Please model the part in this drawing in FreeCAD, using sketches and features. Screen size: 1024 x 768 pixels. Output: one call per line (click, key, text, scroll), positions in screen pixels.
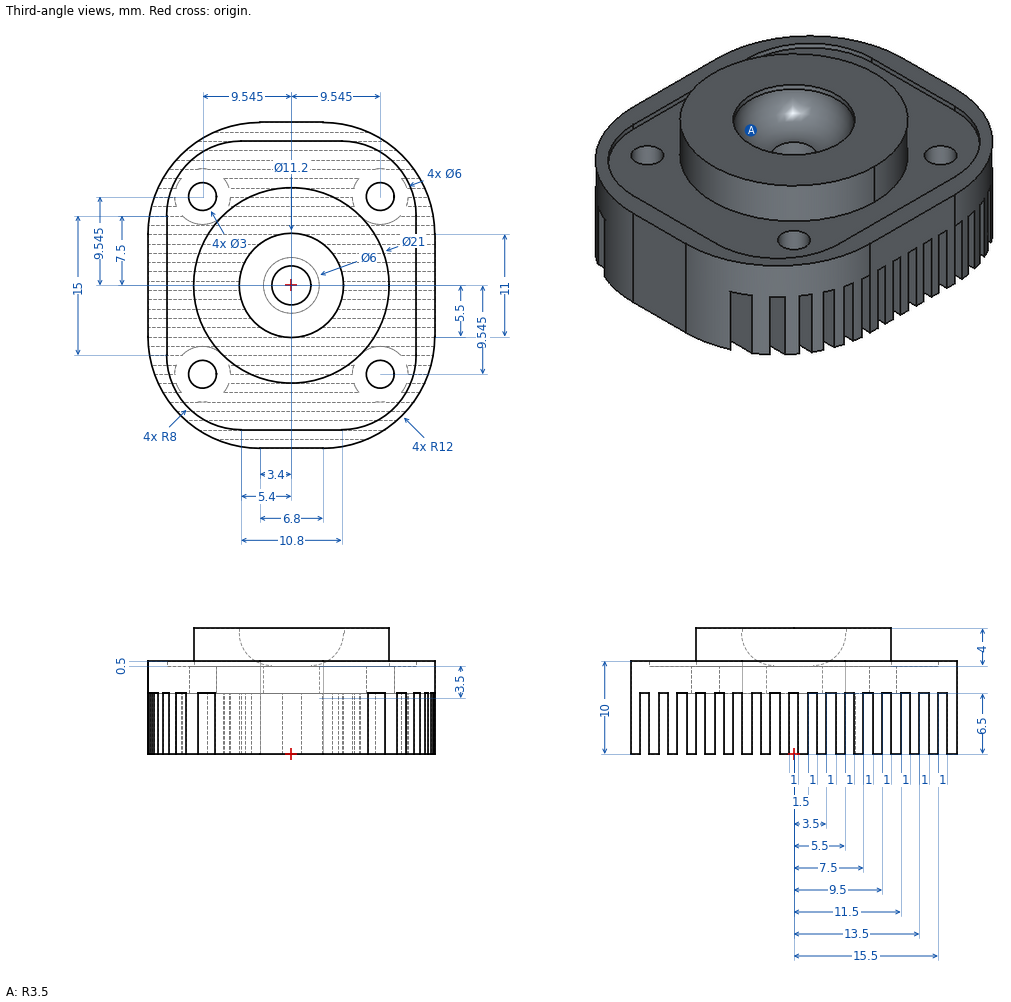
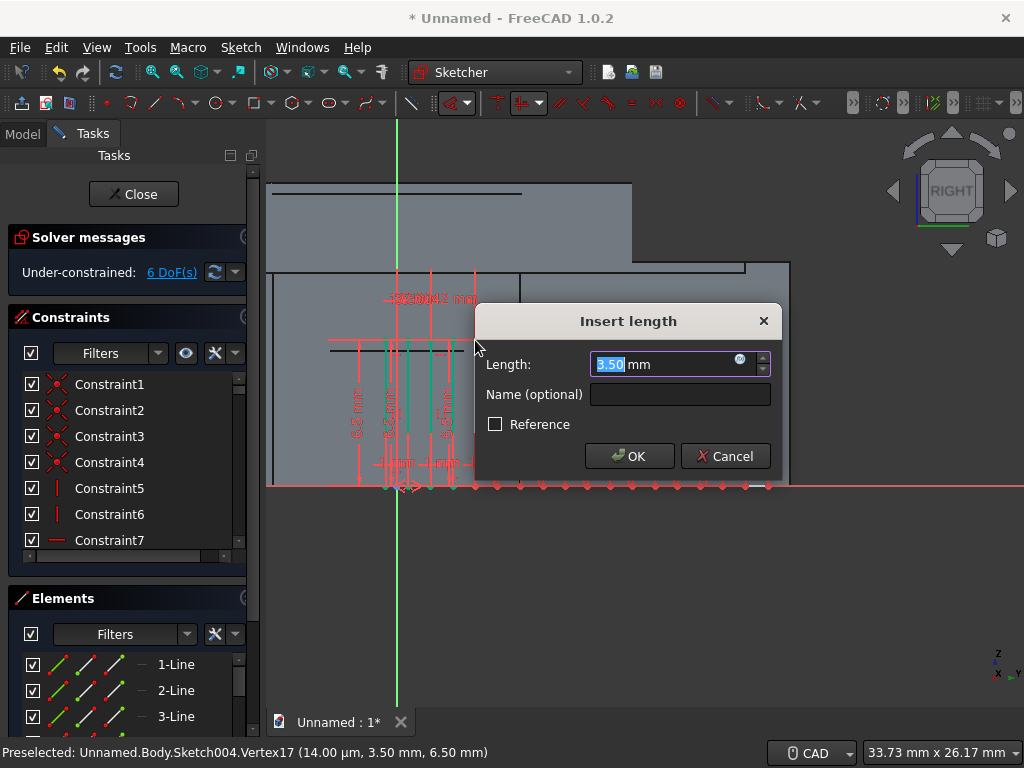
text(3.5)
key(Return)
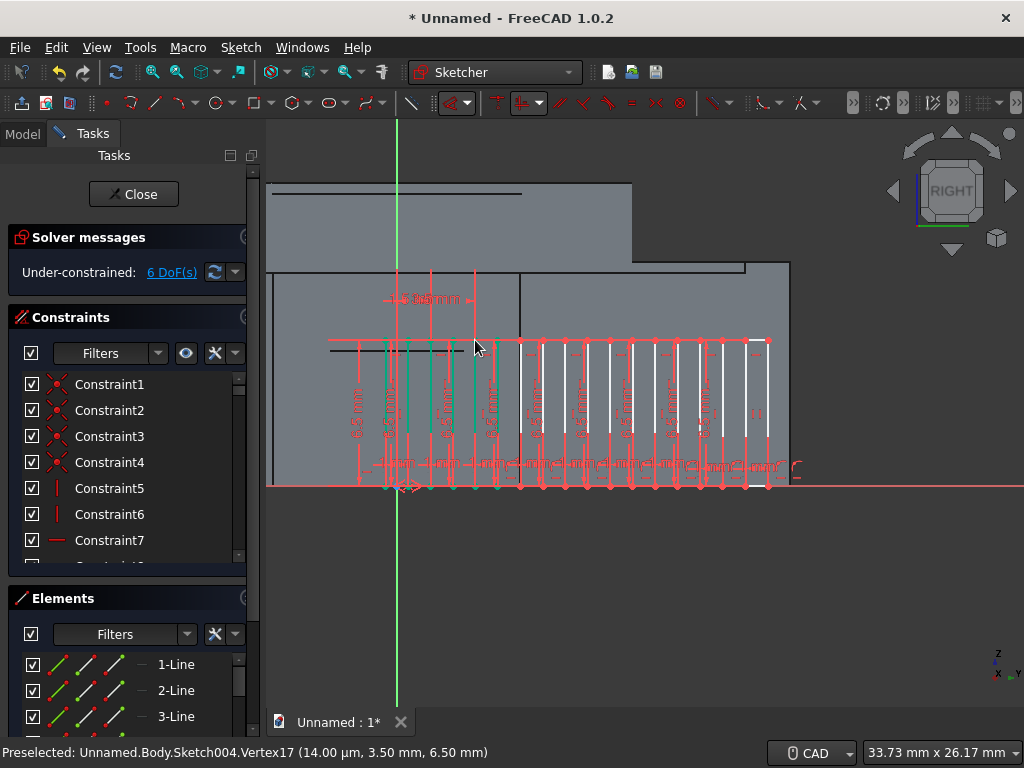
click(521, 340)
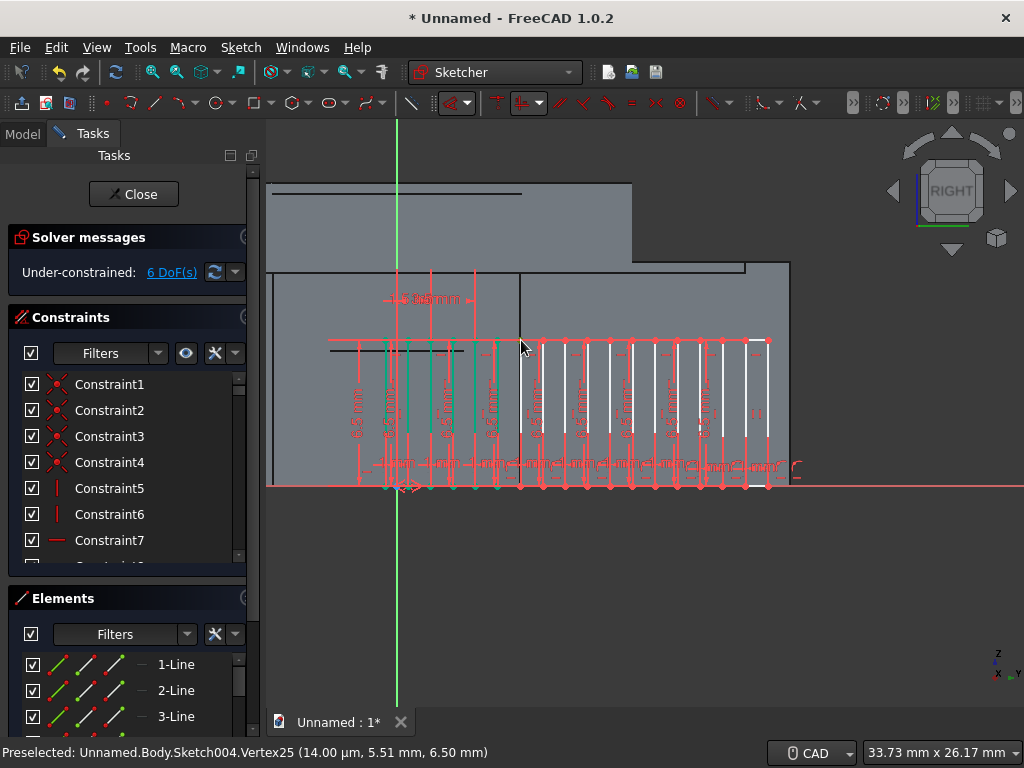
key(l)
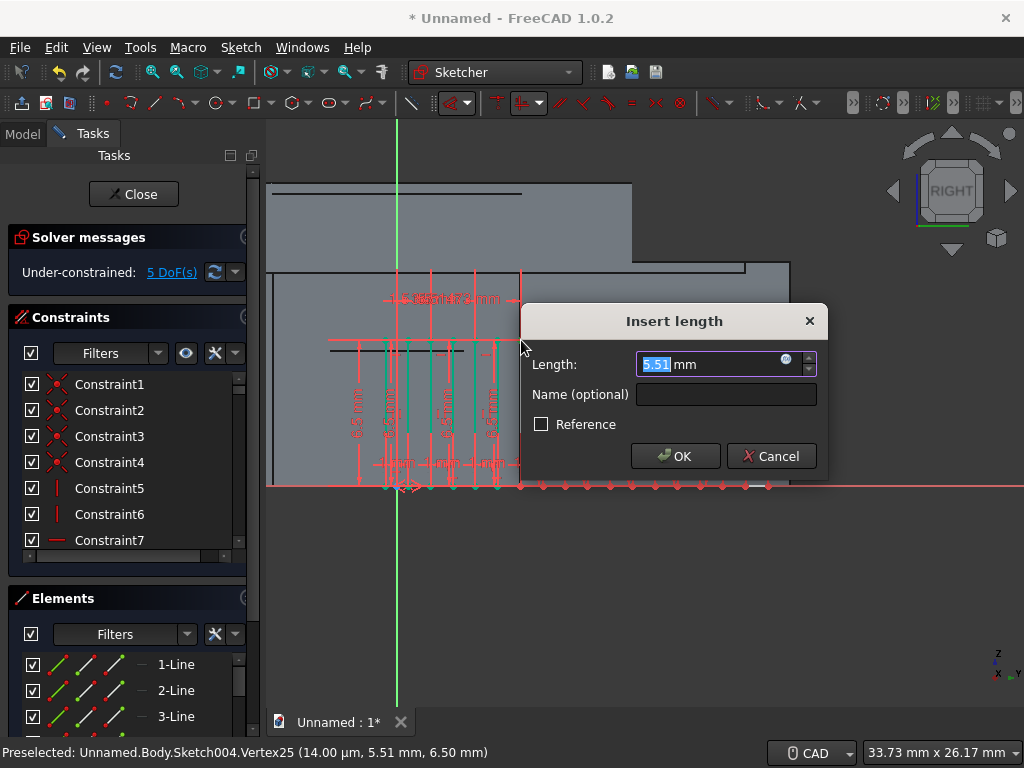
text(5.5)
key(Return)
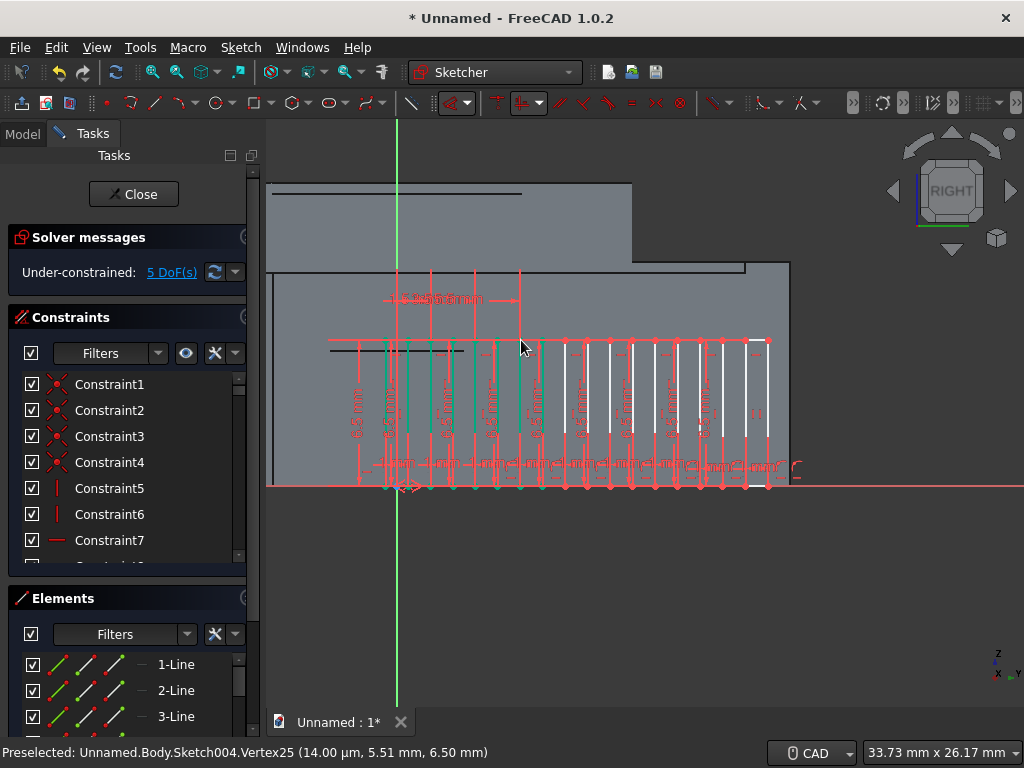
click(565, 340)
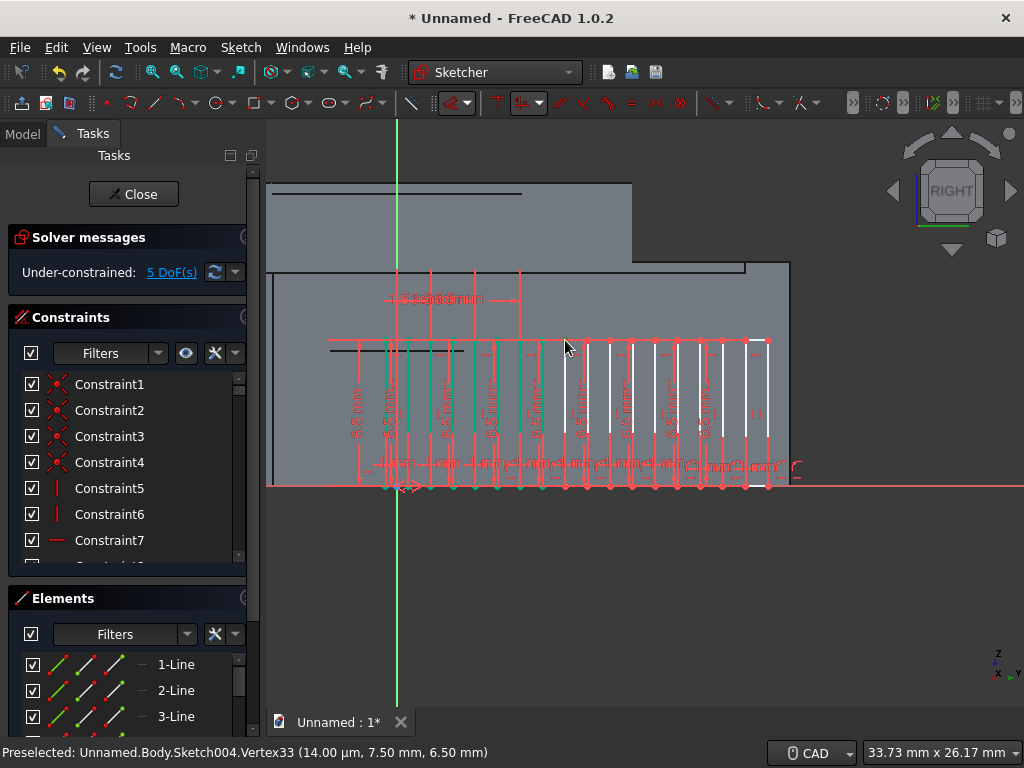
key(l)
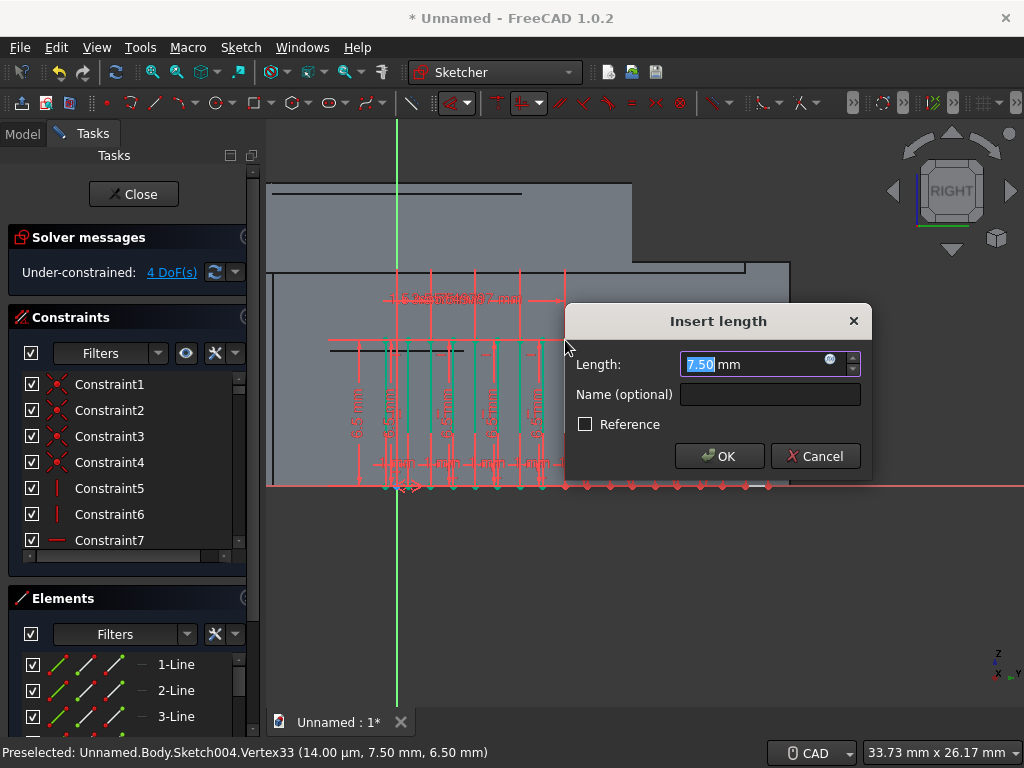
text(7.5)
key(Return)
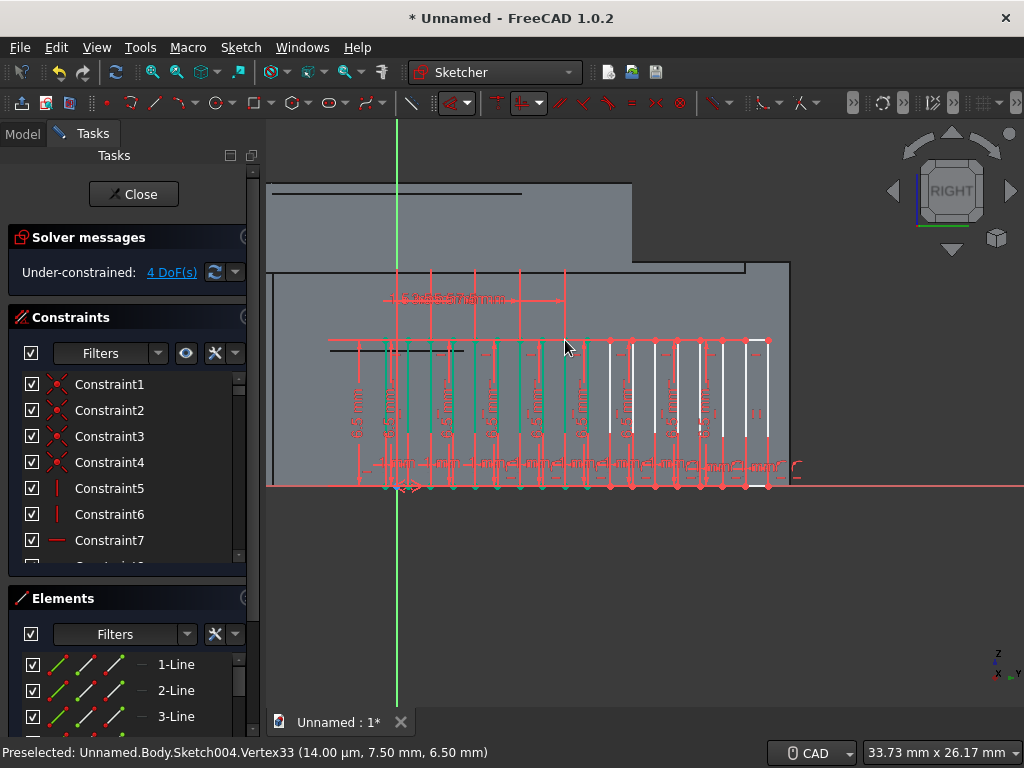
click(610, 340)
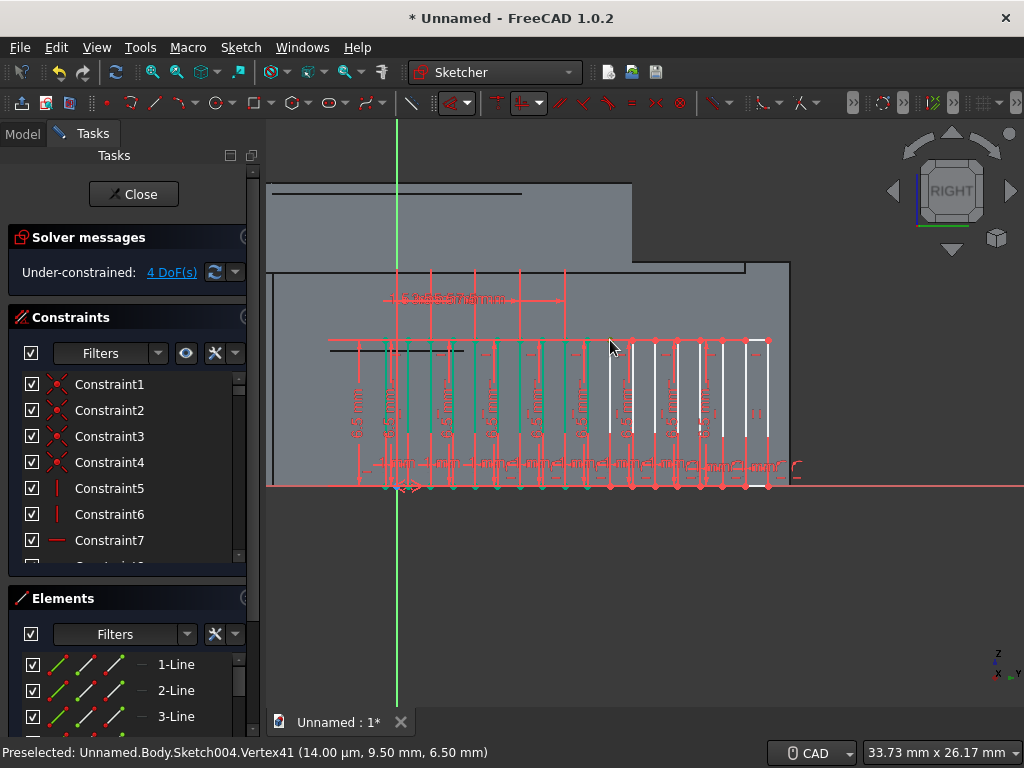
key(l)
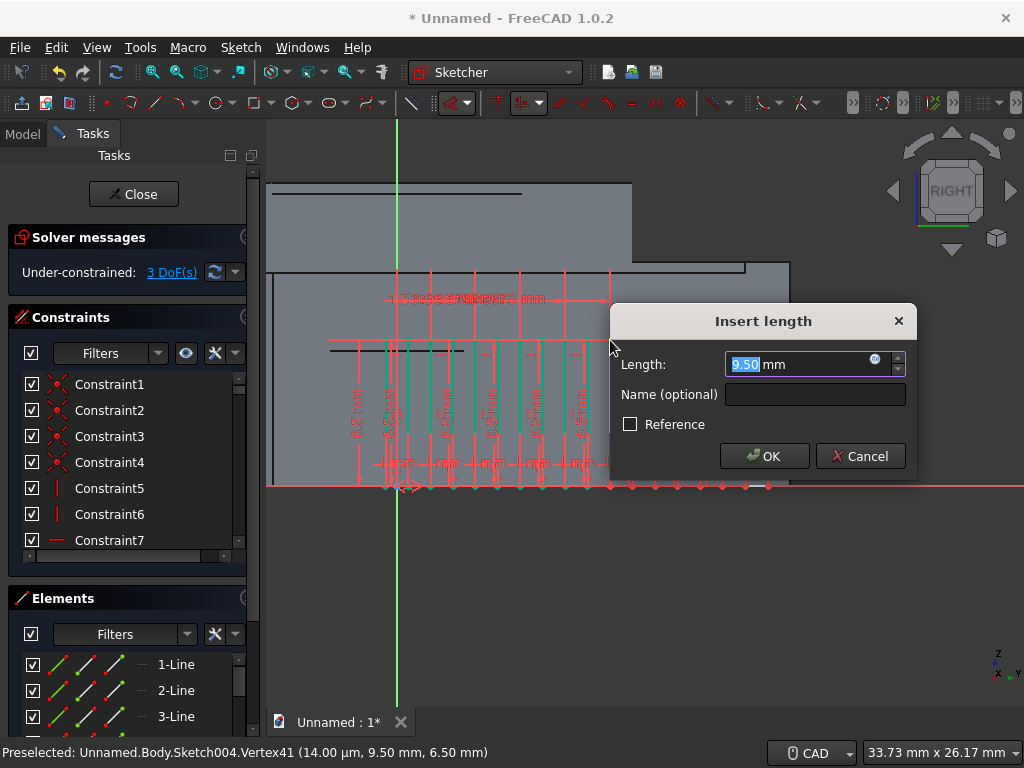
text(9.5)
key(Return)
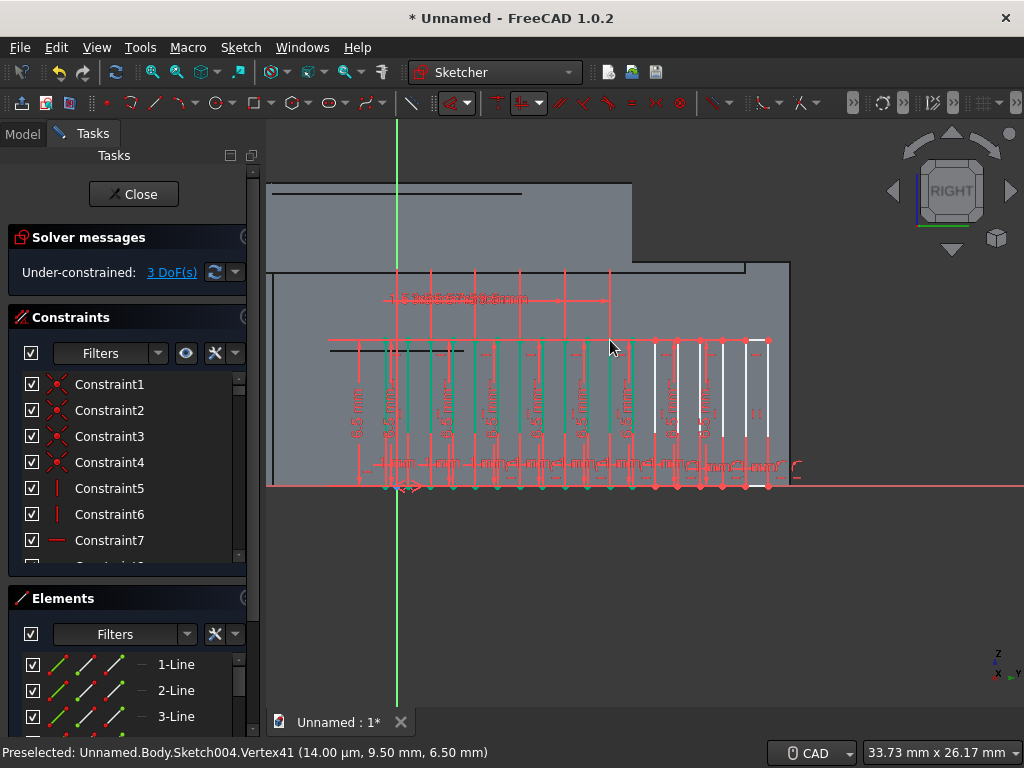
click(655, 340)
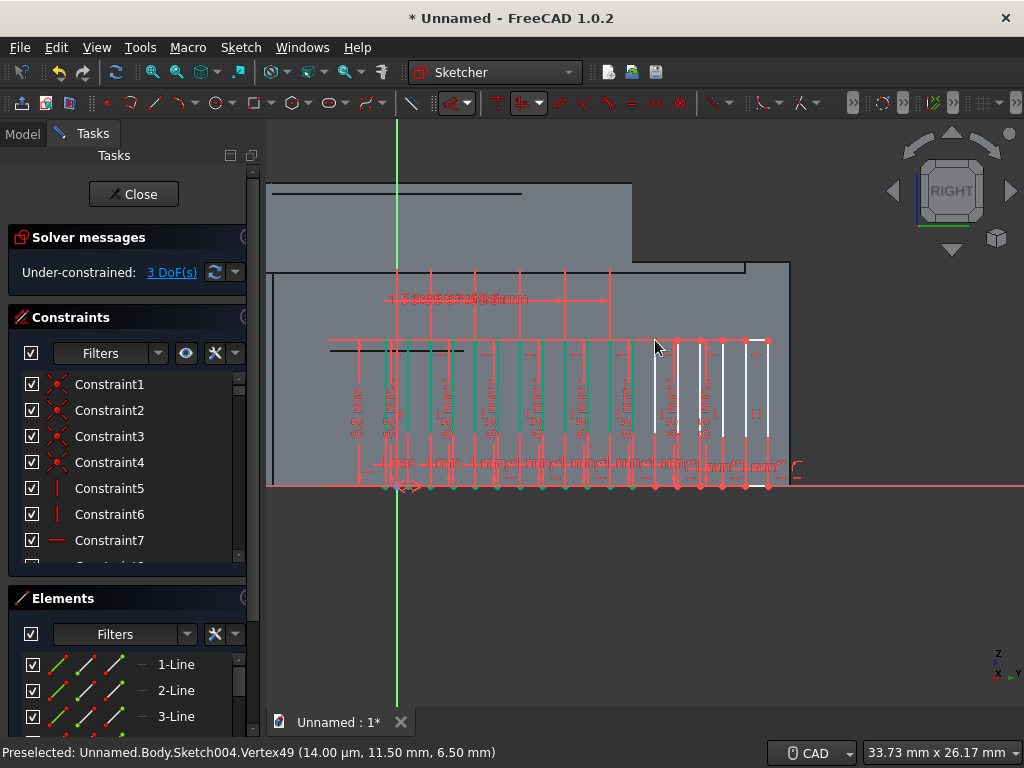
key(l)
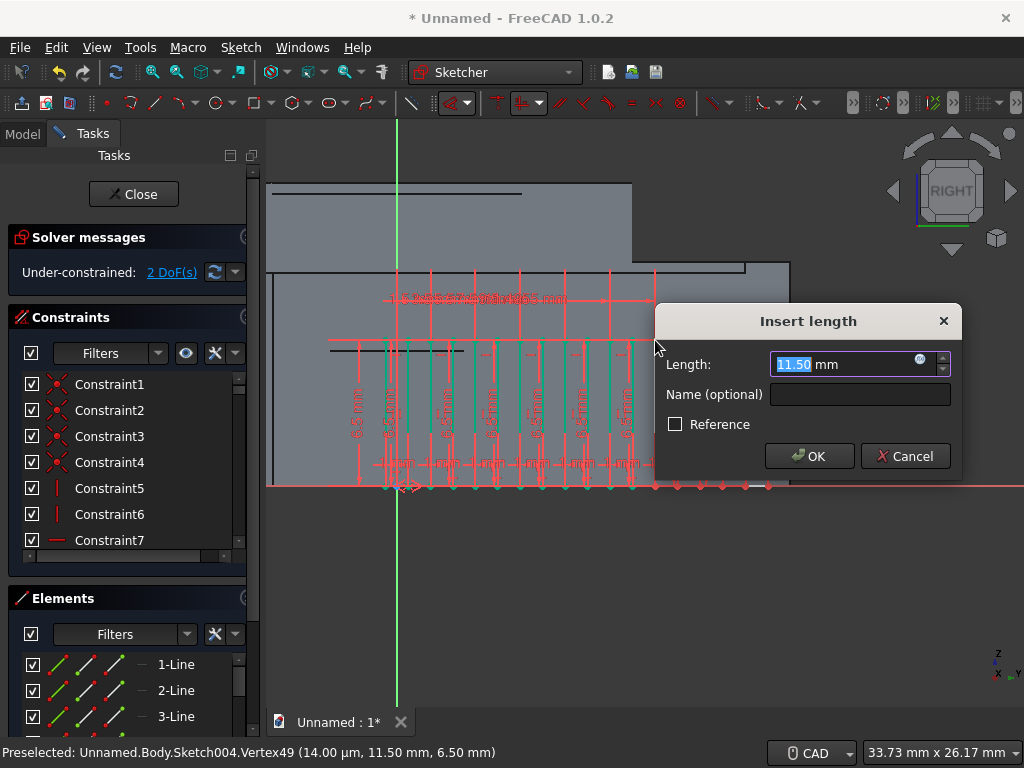
text(11.5)
key(Return)